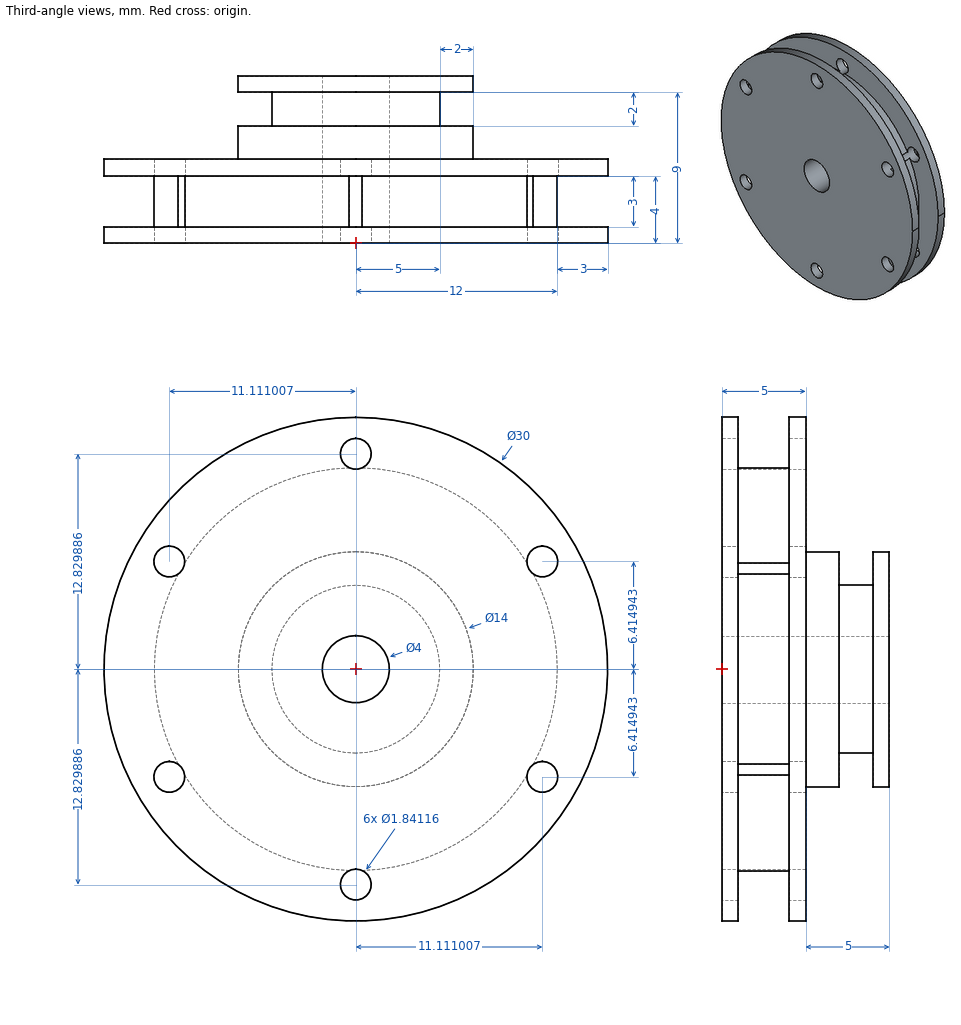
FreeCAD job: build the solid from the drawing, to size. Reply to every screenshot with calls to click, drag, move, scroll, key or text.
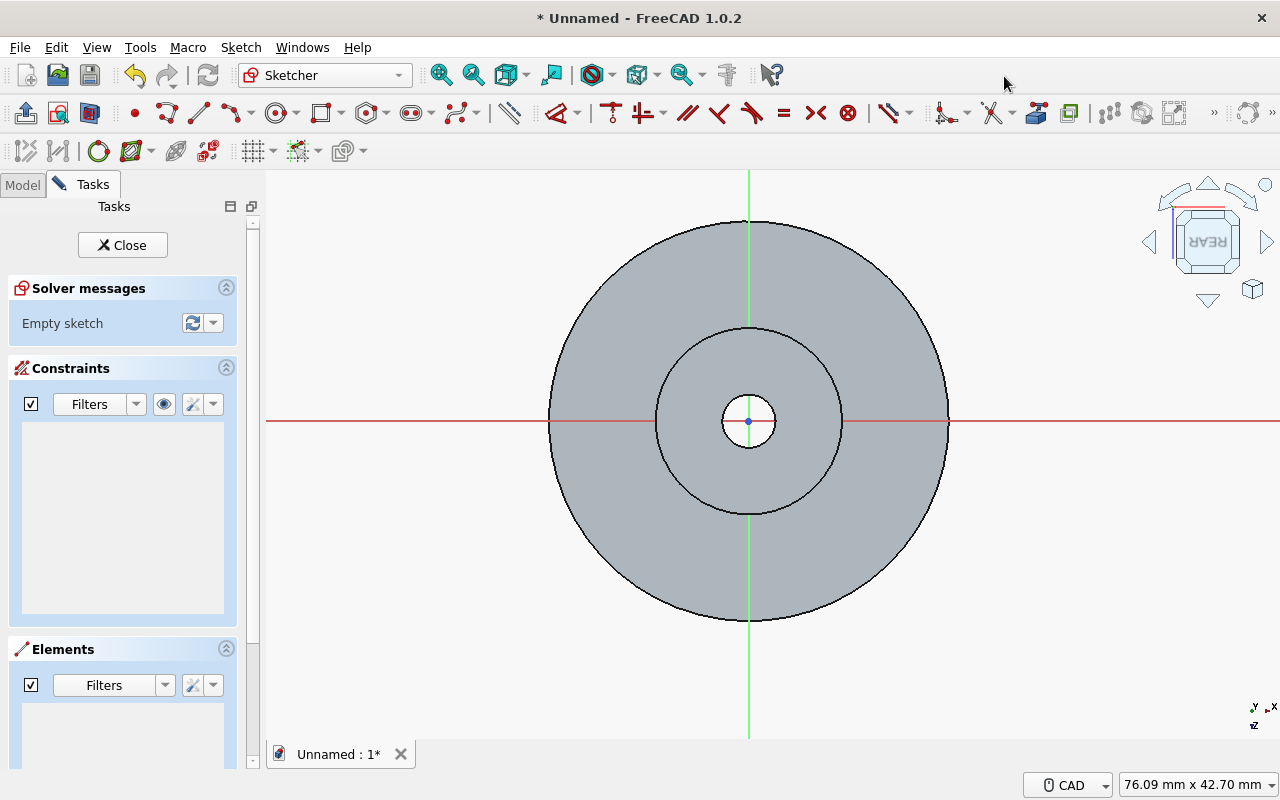
click(90, 114)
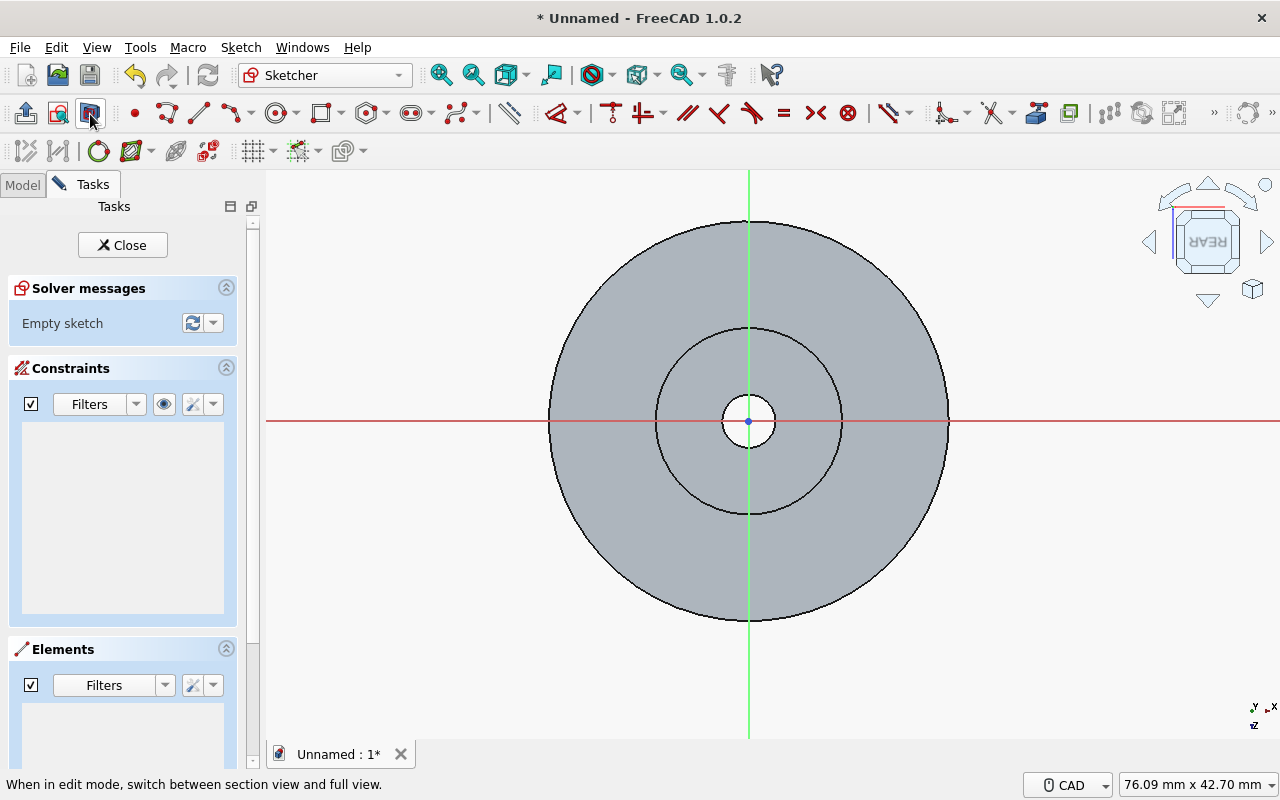
click(276, 114)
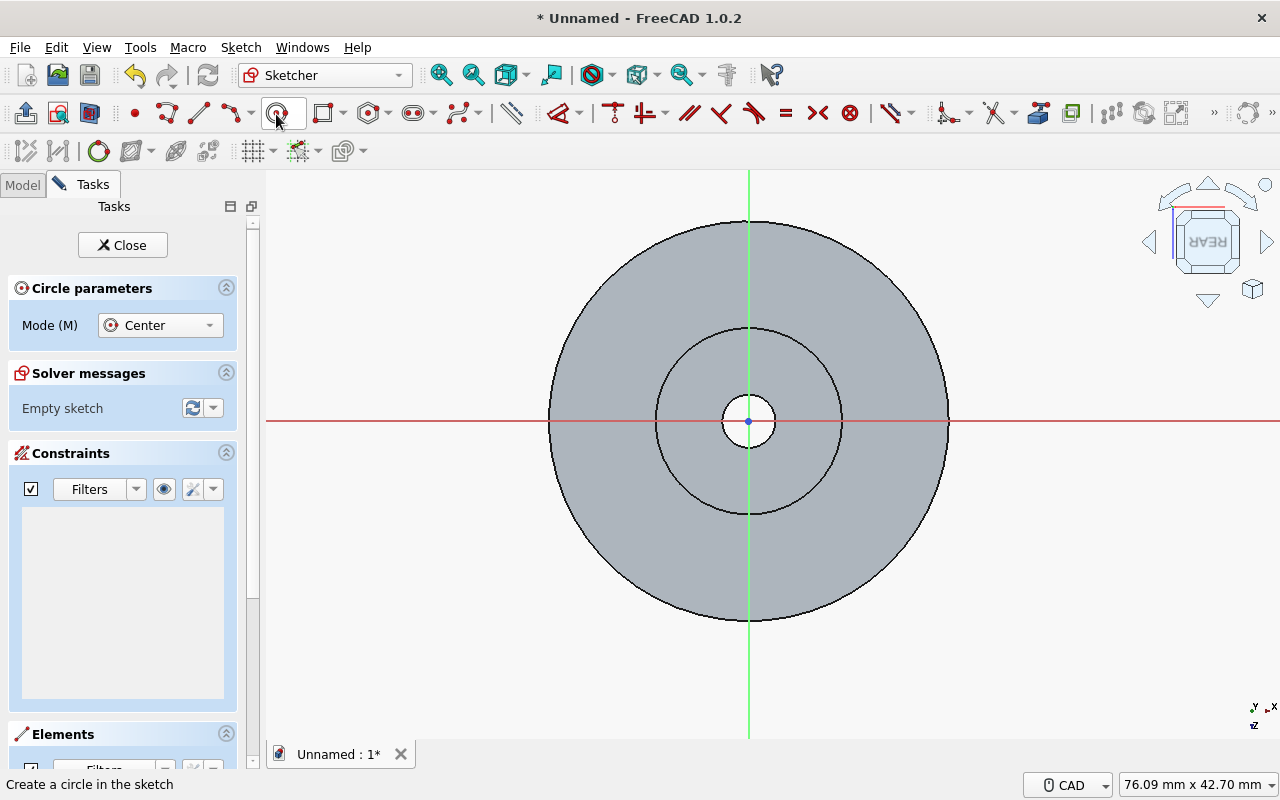
scroll(749, 250, up, 4)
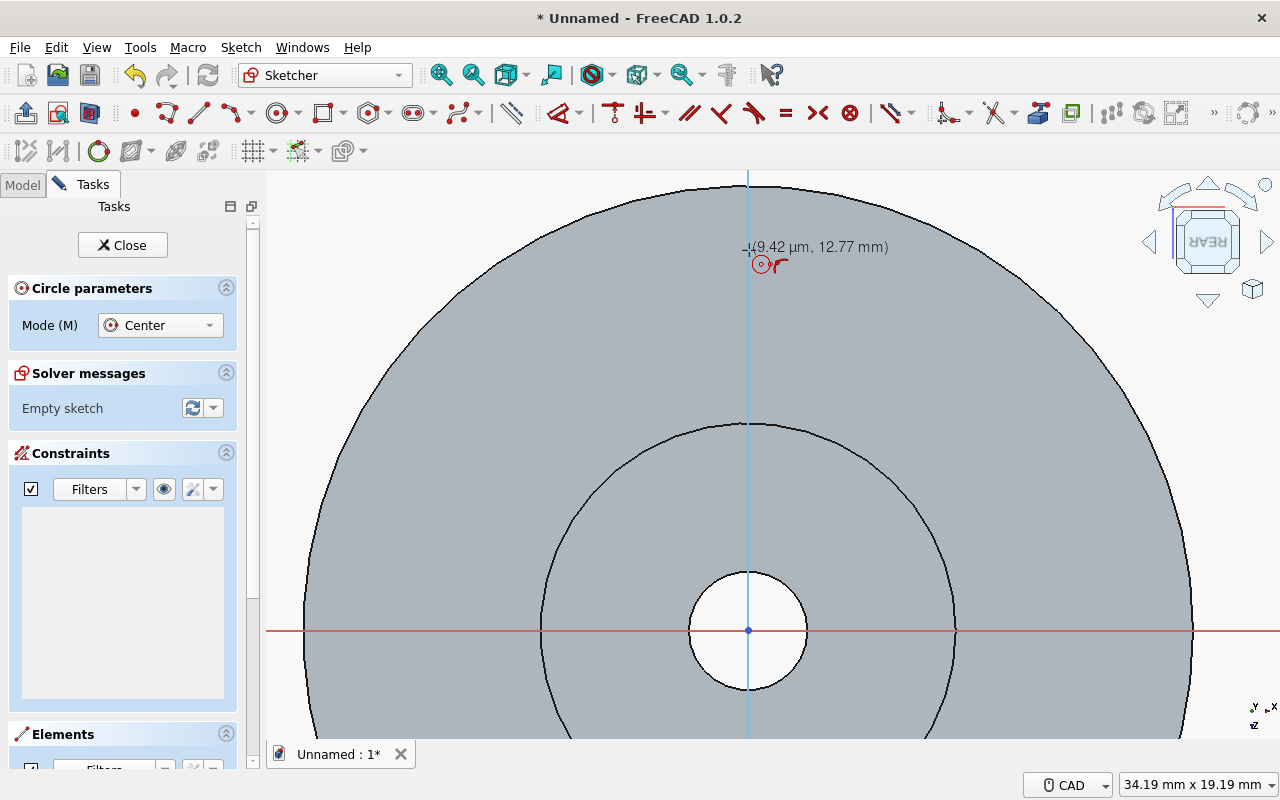
click(748, 250)
move(767, 231)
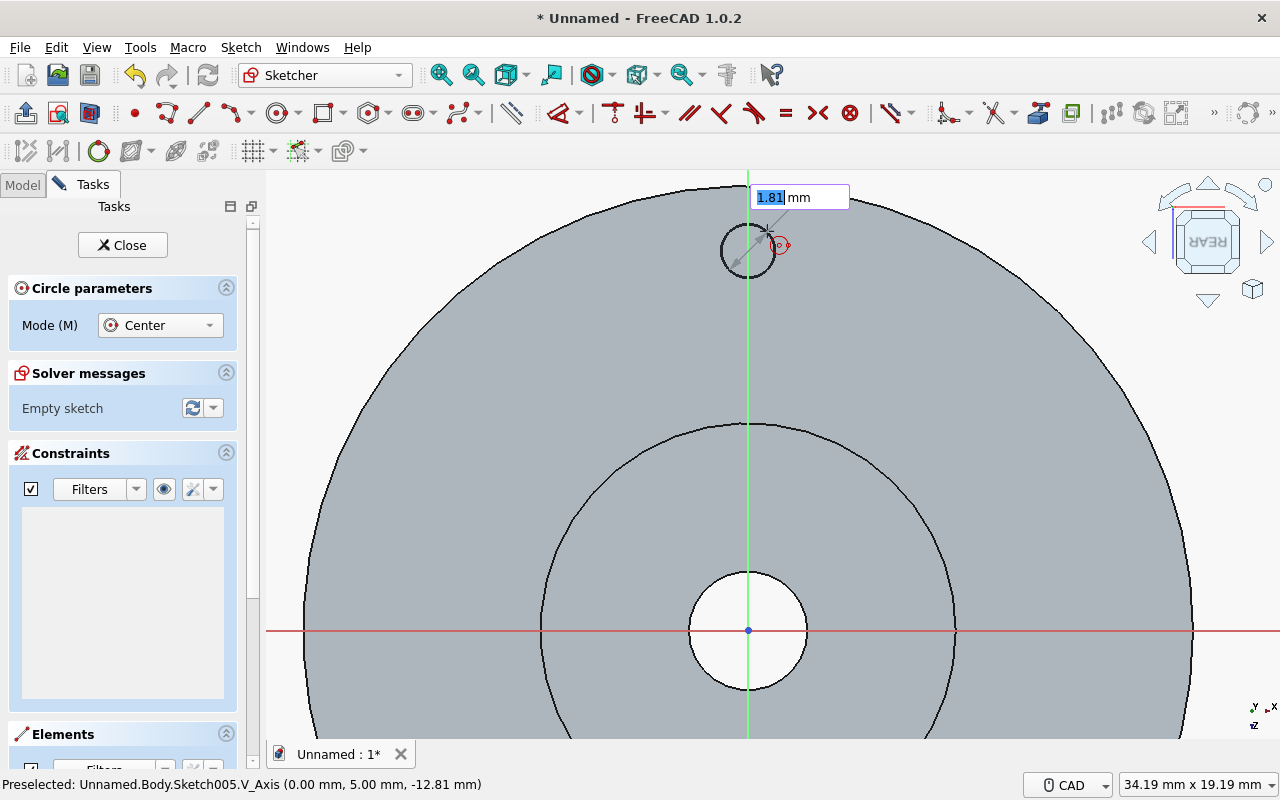
text(1.84116)
key(Return)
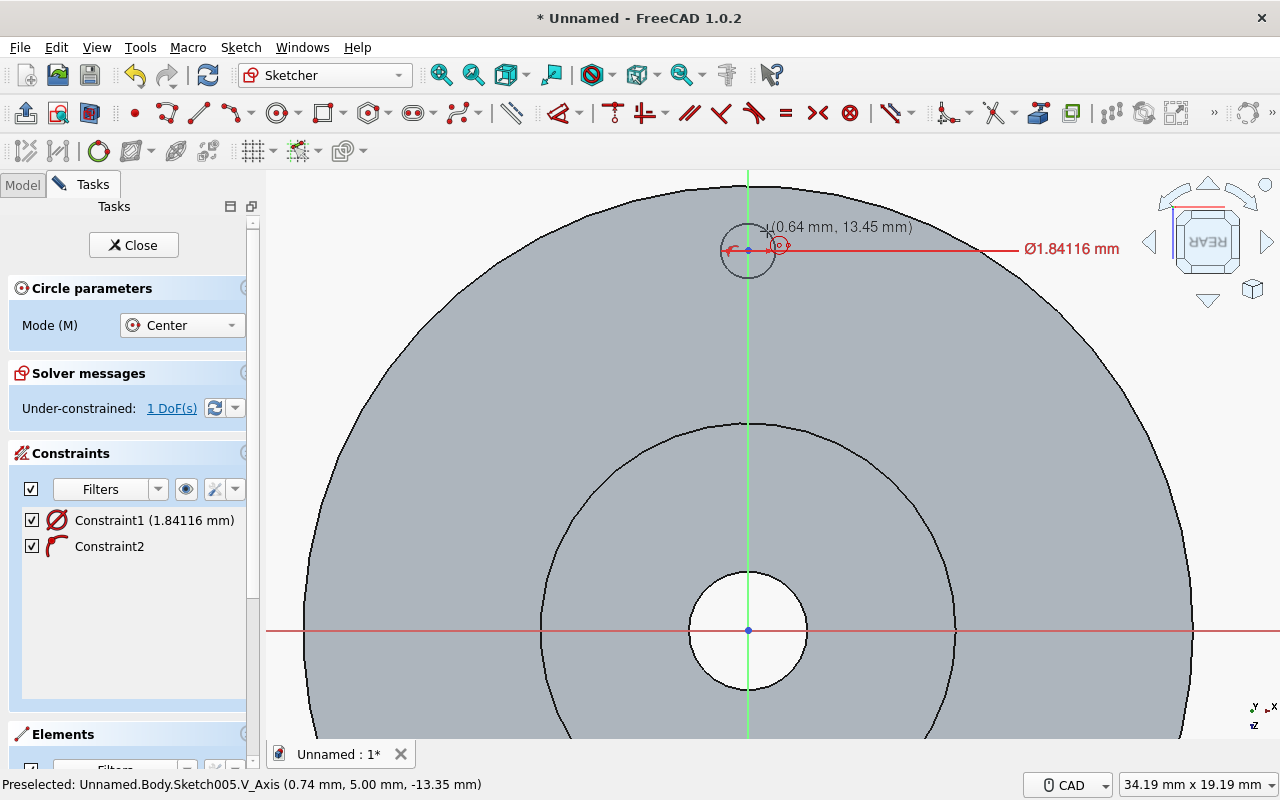
click(1078, 441)
move(1097, 421)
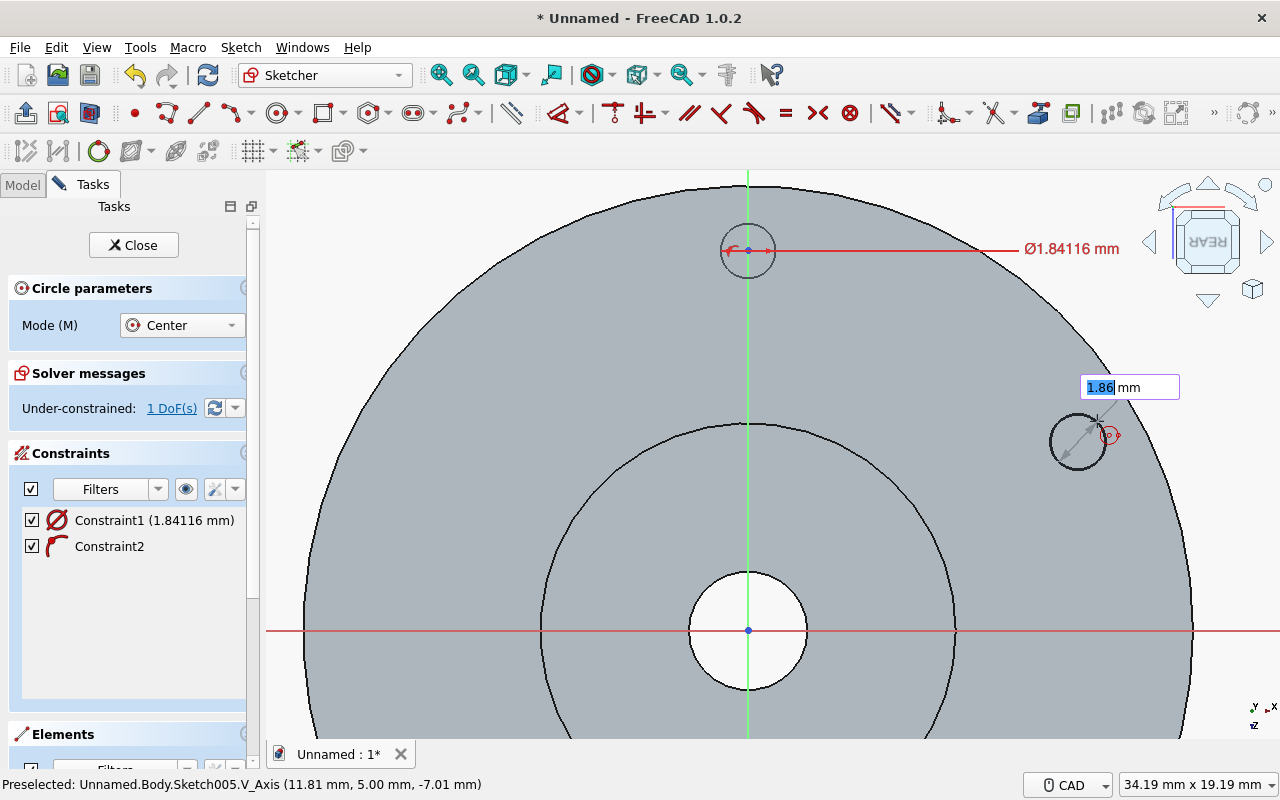
text(1.84116)
key(Return)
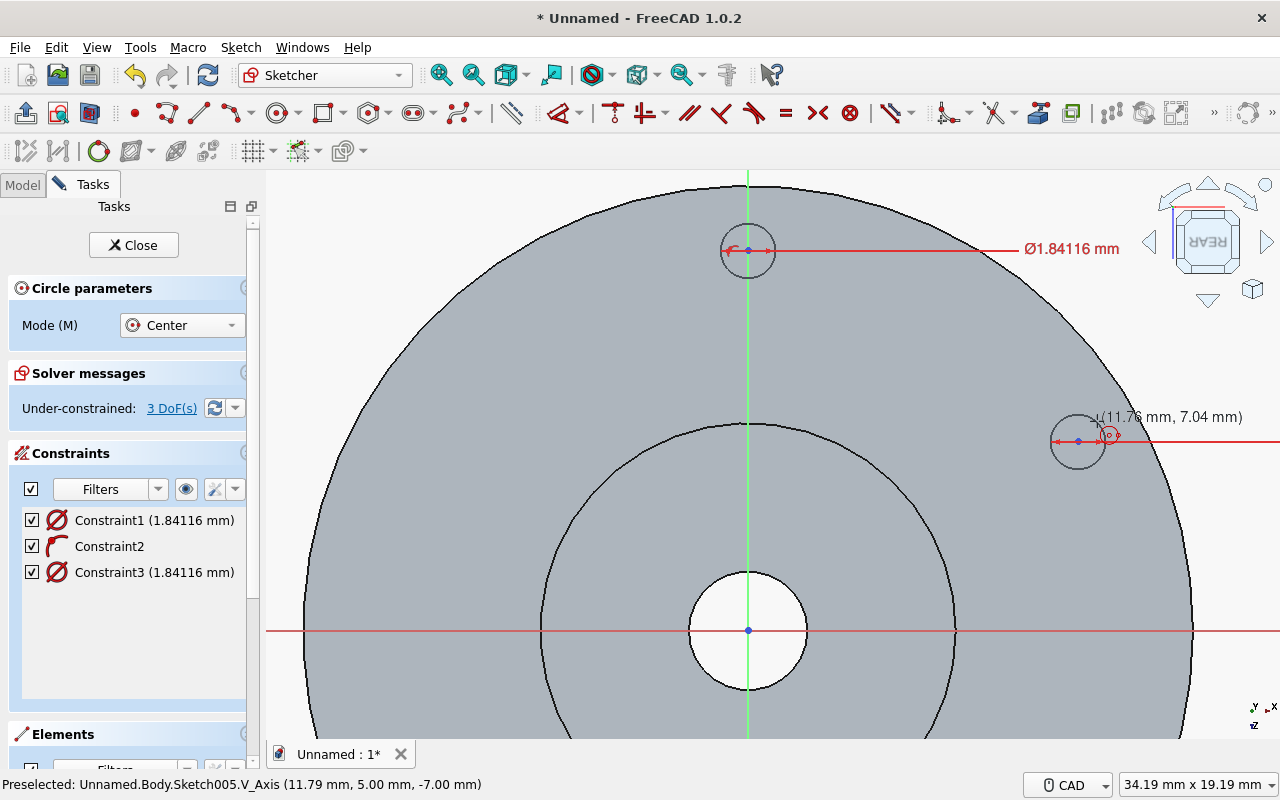
scroll(669, 311, down, 4)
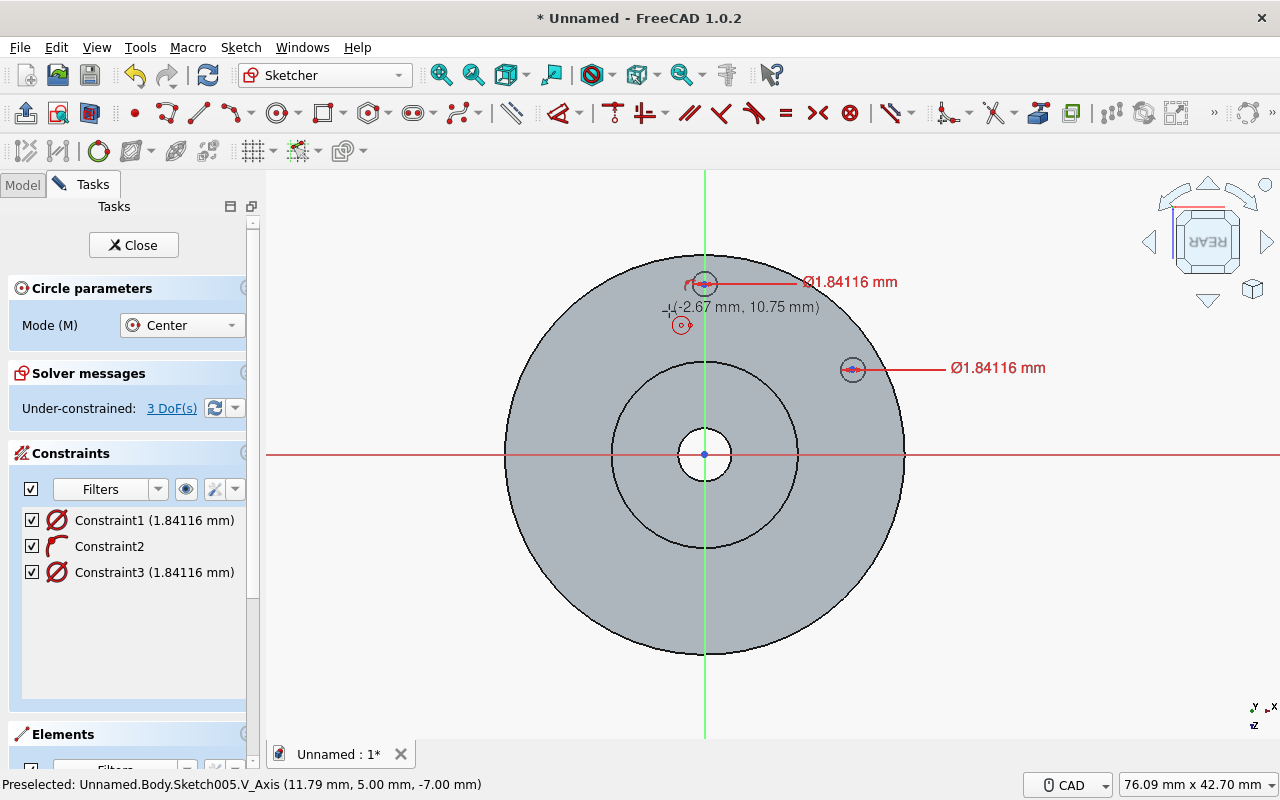
scroll(853, 540, up, 4)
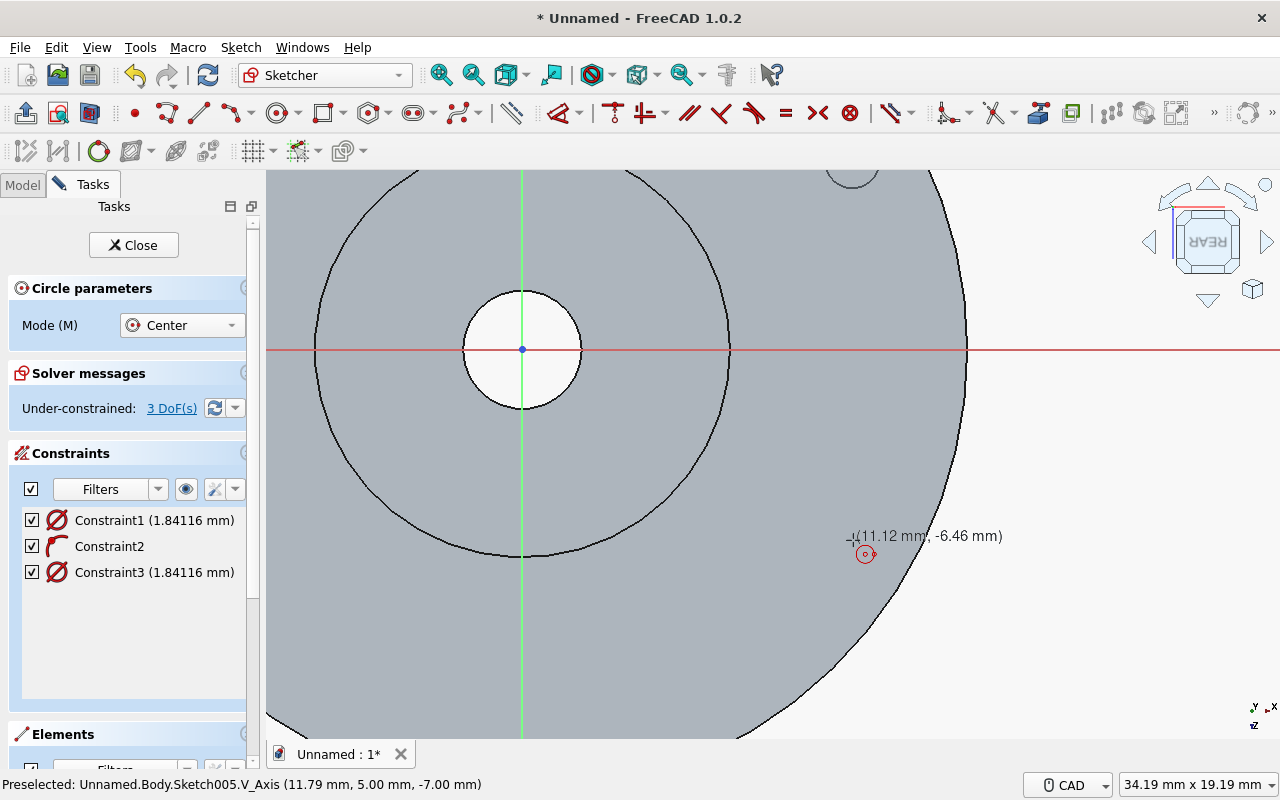
click(852, 540)
move(871, 521)